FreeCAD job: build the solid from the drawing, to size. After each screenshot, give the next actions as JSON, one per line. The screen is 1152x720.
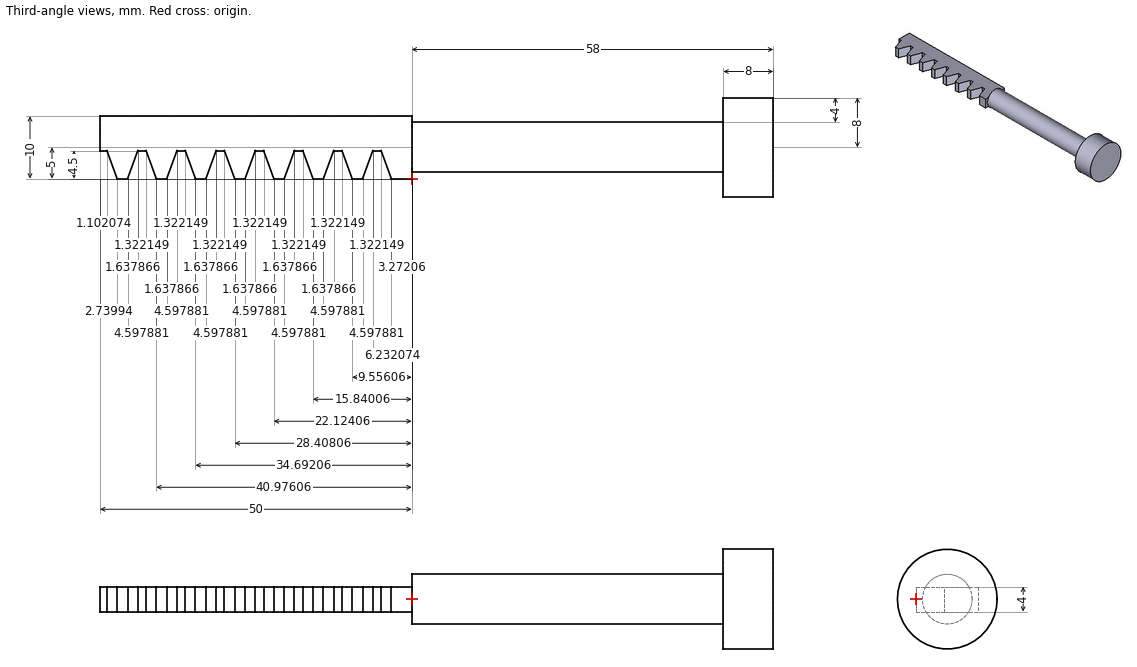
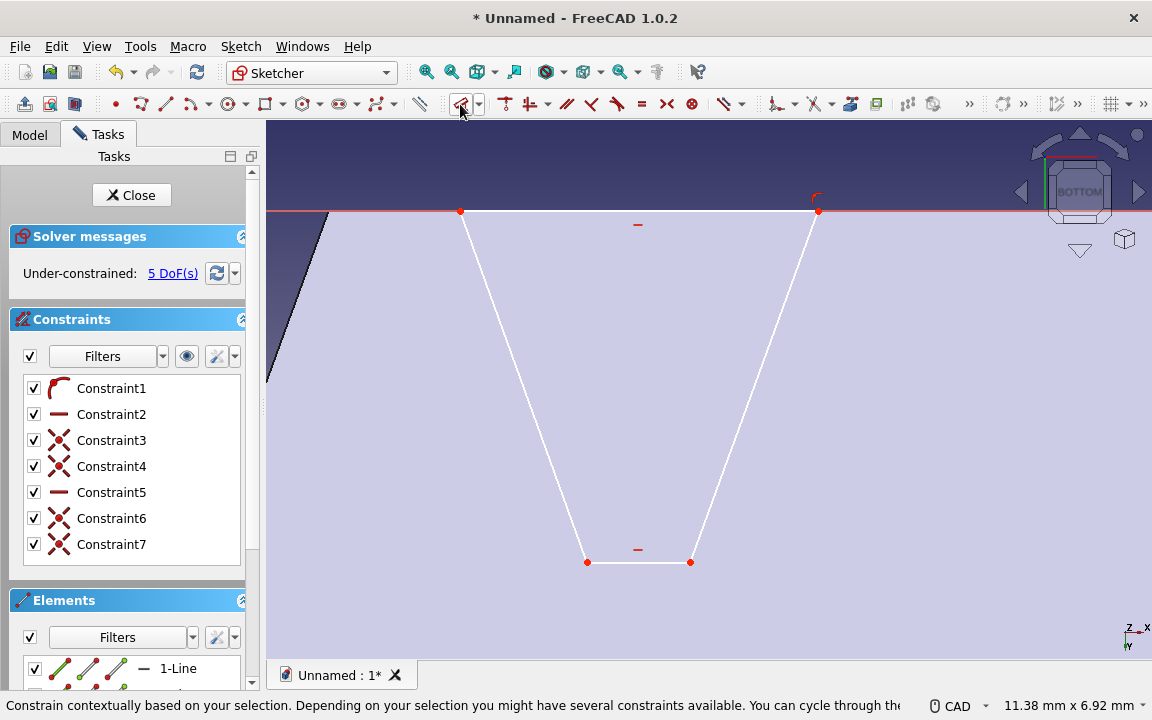
{"action": "left_click", "coordinate": [587, 563]}
{"action": "left_click", "coordinate": [553, 387]}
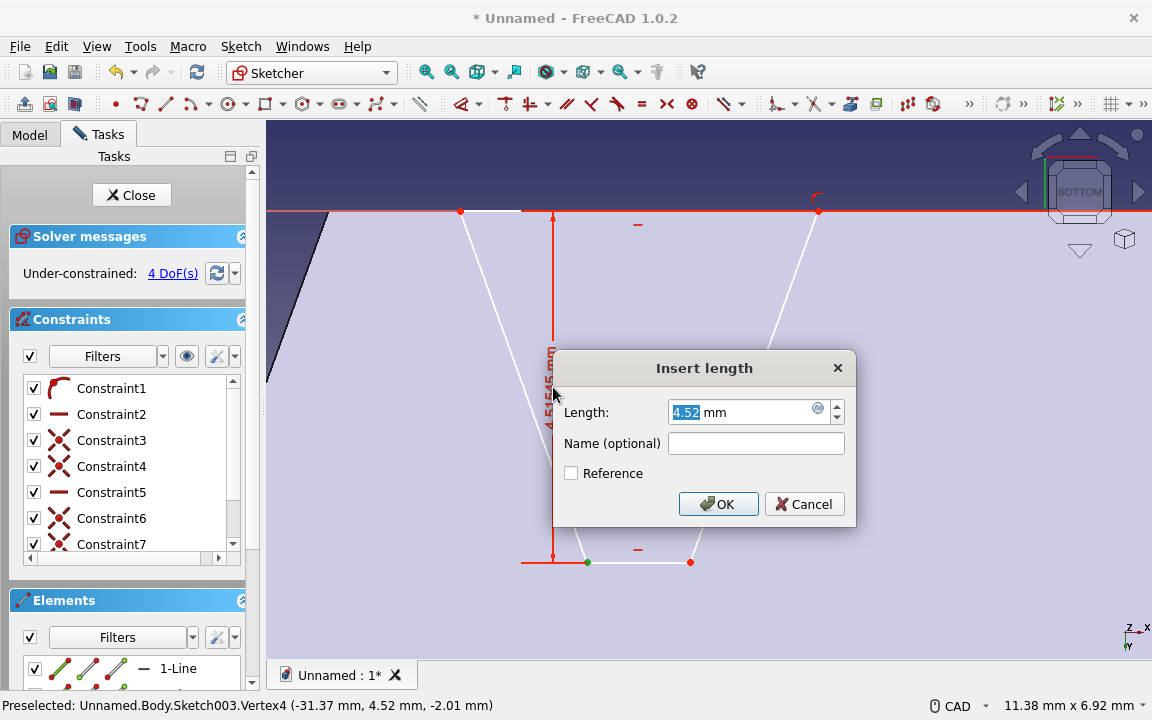
{"action": "type", "text": "4.5"}
{"action": "key", "text": "Return"}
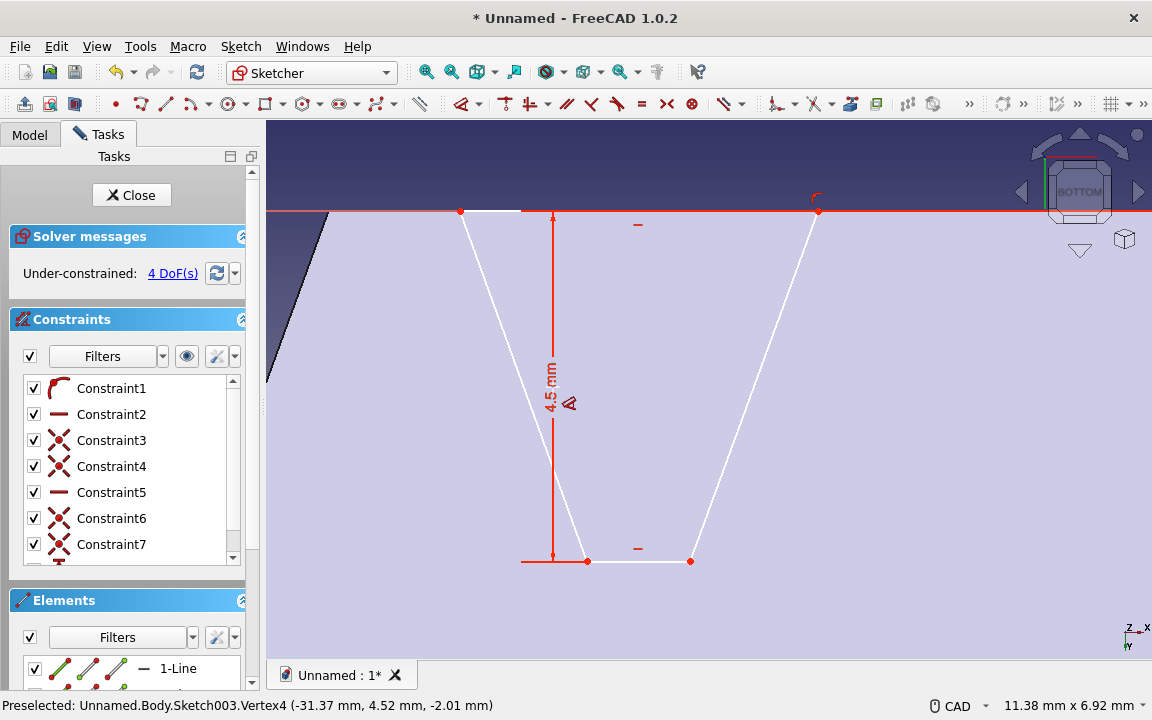
{"action": "left_click", "coordinate": [711, 211]}
{"action": "left_click", "coordinate": [639, 177]}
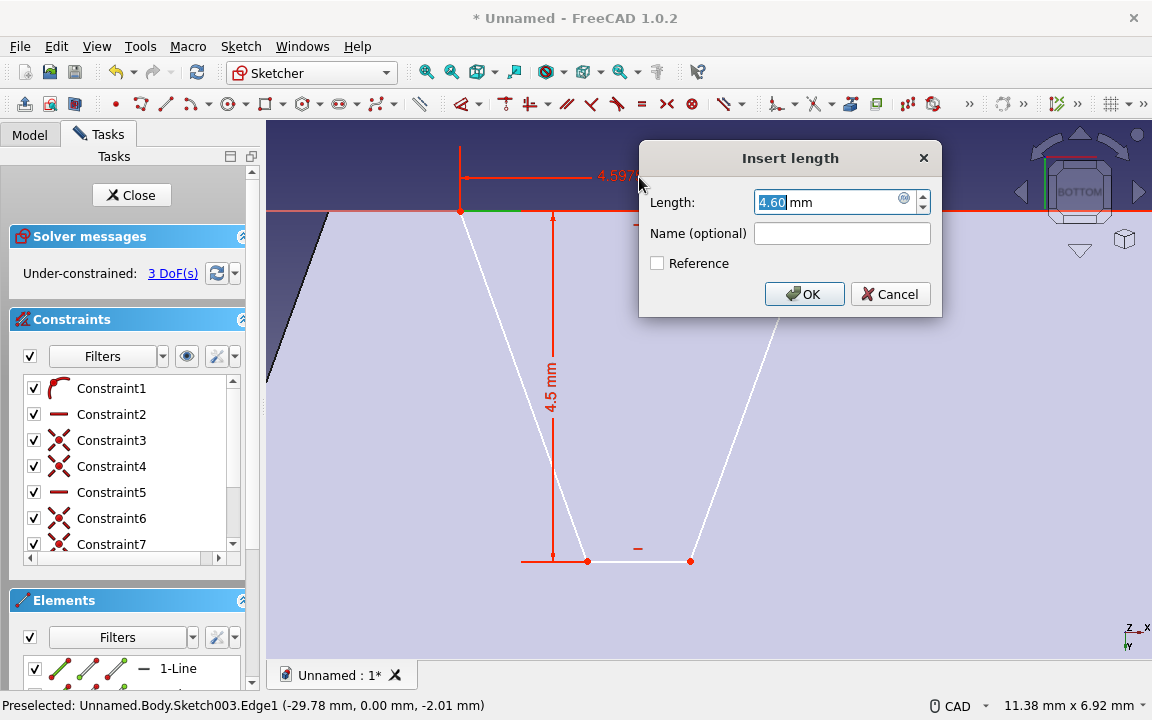
{"action": "type", "text": "4.597881"}
{"action": "key", "text": "Return"}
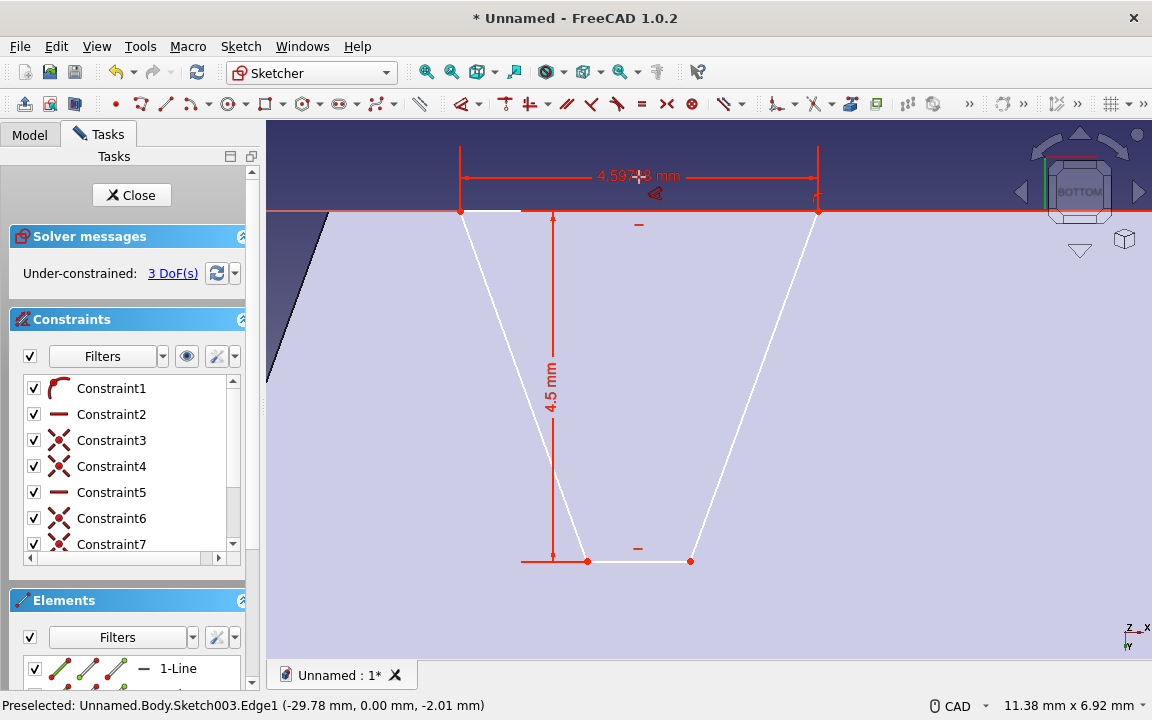
{"action": "left_click", "coordinate": [618, 562]}
{"action": "left_click", "coordinate": [638, 596]}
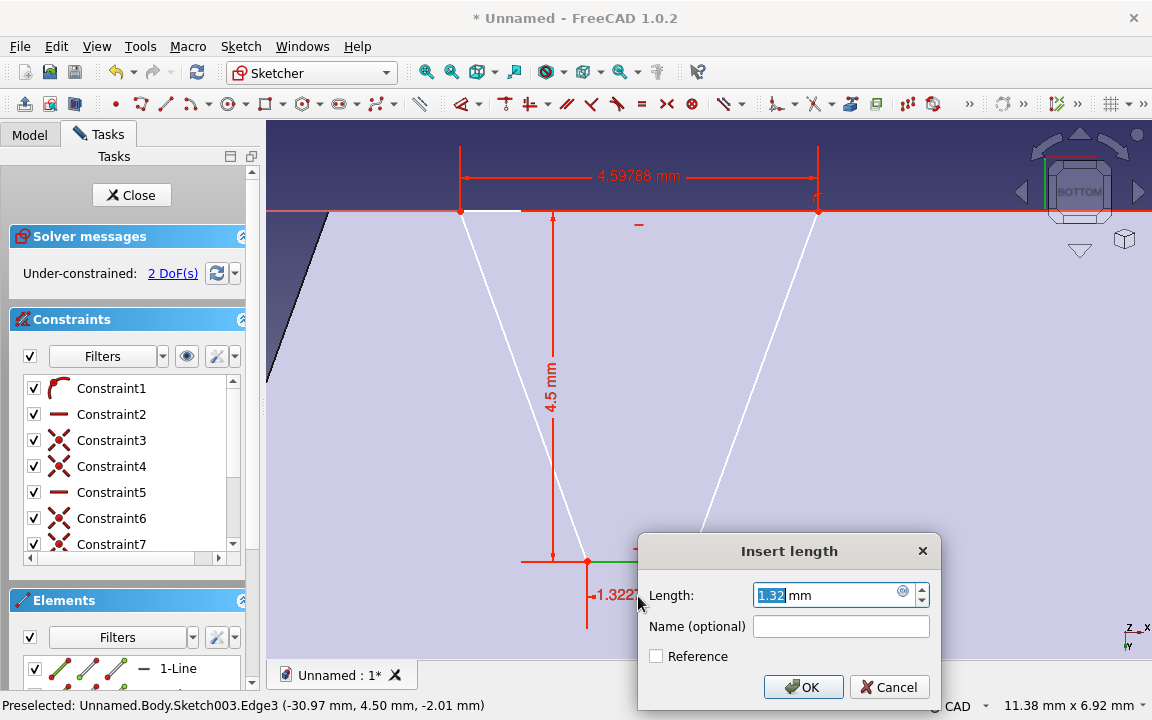
{"action": "type", "text": "1.322149"}
{"action": "key", "text": "Return"}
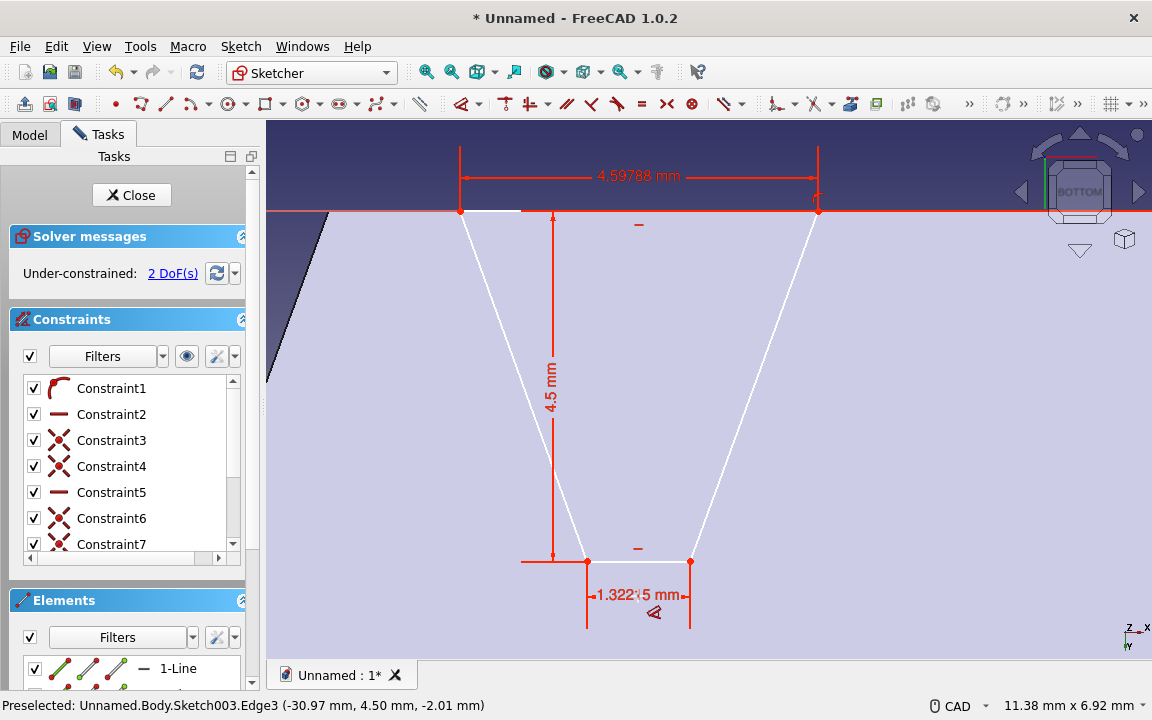
{"action": "left_click", "coordinate": [818, 211]}
{"action": "left_click", "coordinate": [903, 177]}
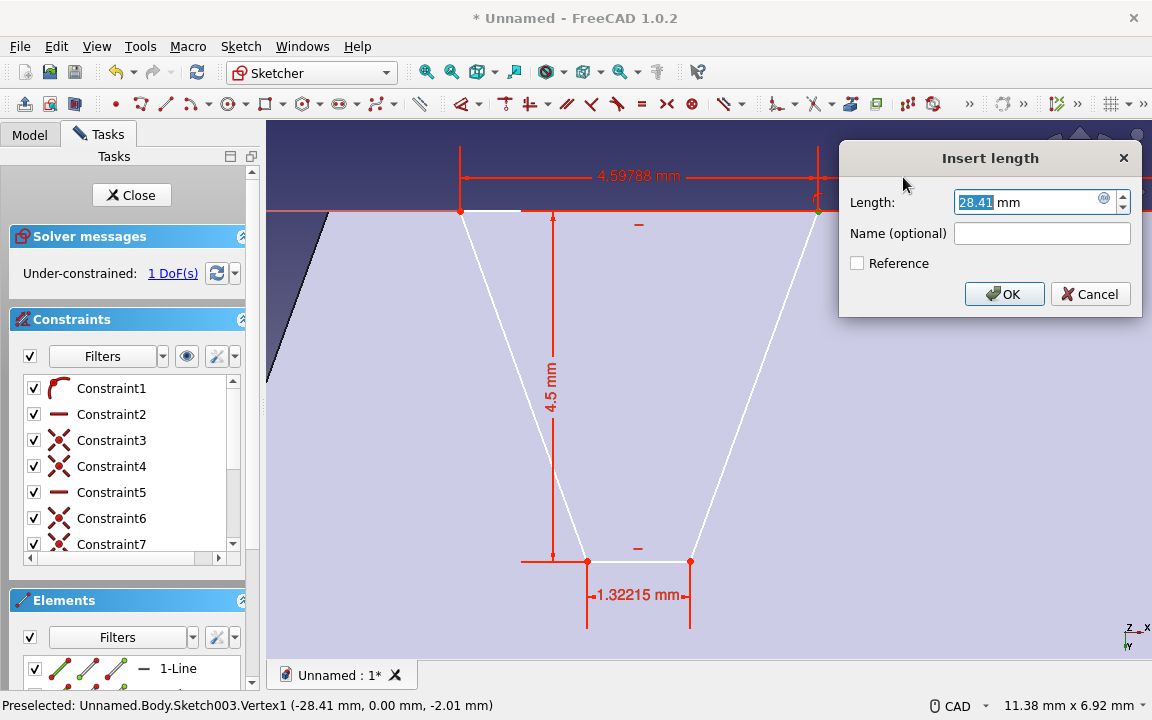
{"action": "type", "text": "28.40806"}
{"action": "key", "text": "Return"}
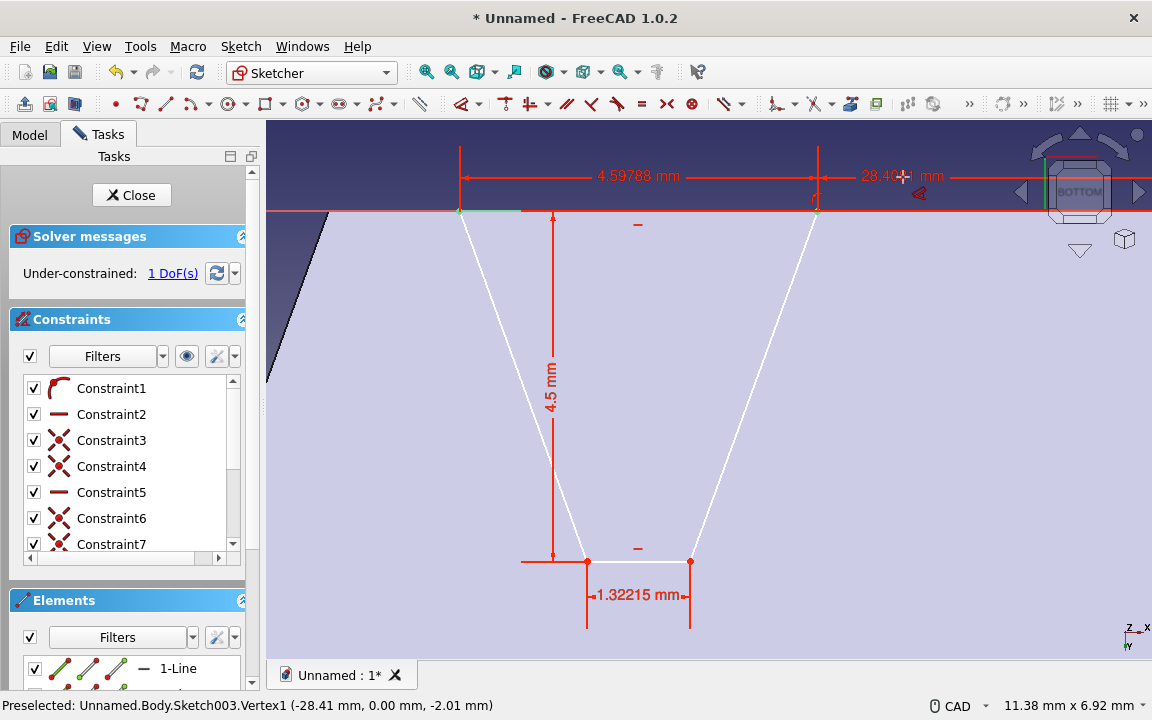
{"action": "left_click", "coordinate": [498, 317]}
{"action": "left_click", "coordinate": [523, 596]}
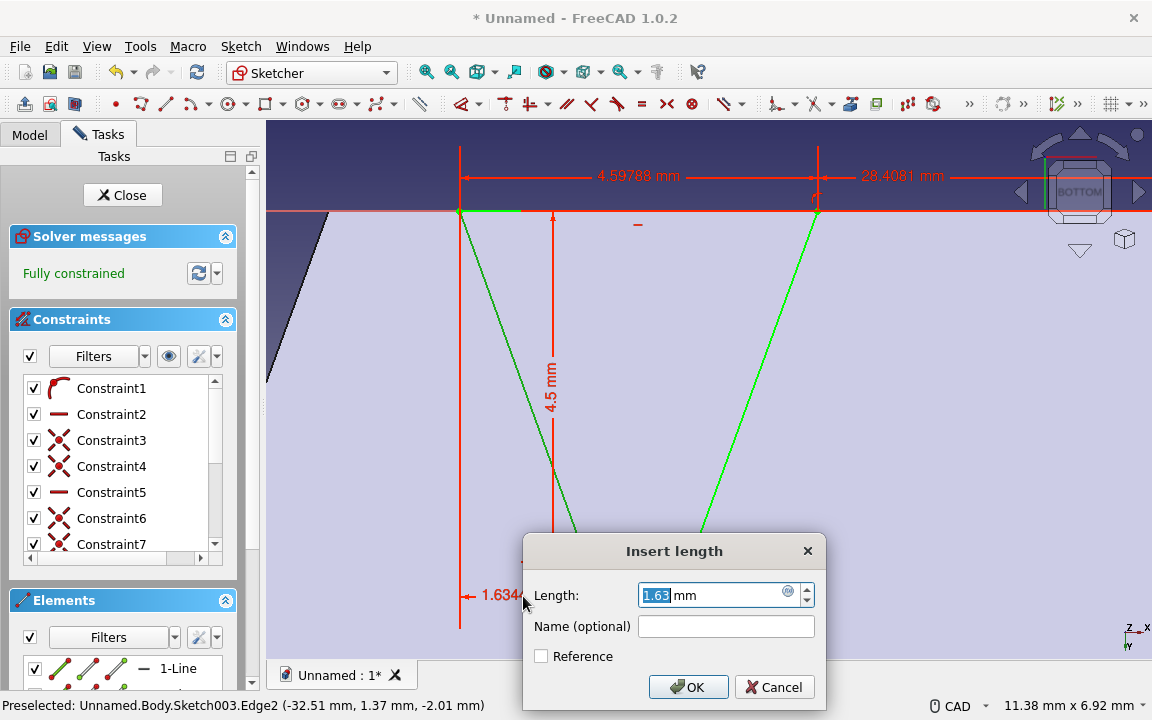
{"action": "type", "text": "1.637866"}
{"action": "key", "text": "Return"}
{"action": "key", "text": "Escape"}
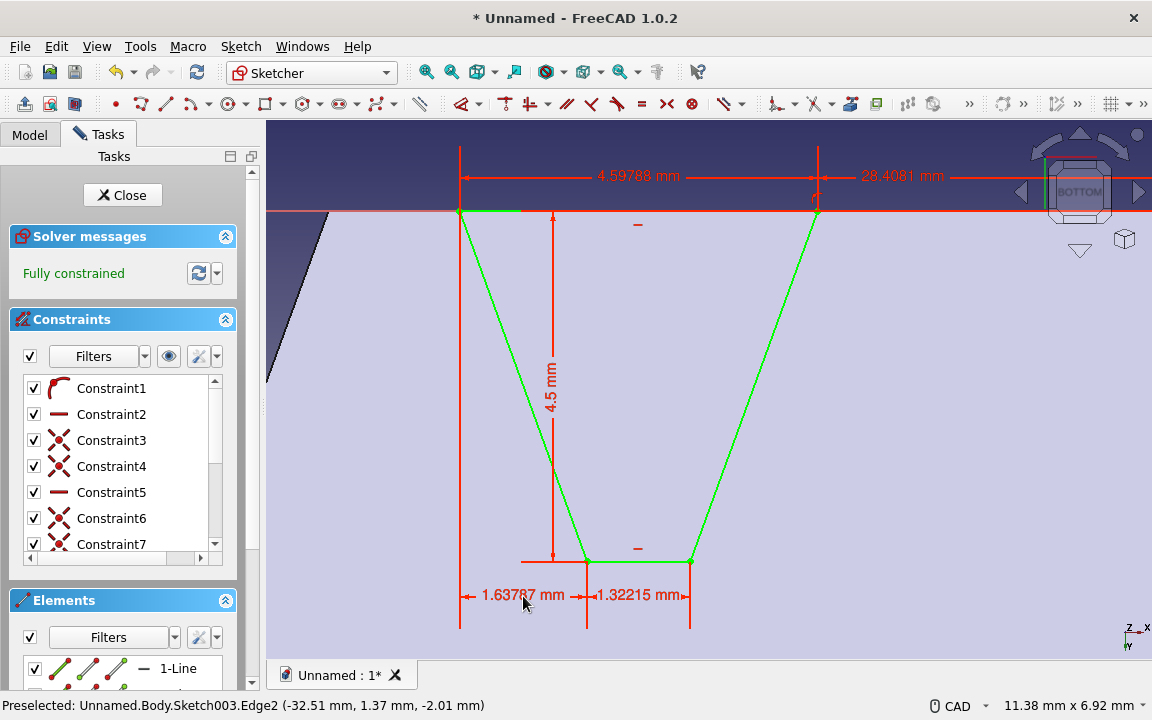
{"action": "left_click", "coordinate": [123, 195]}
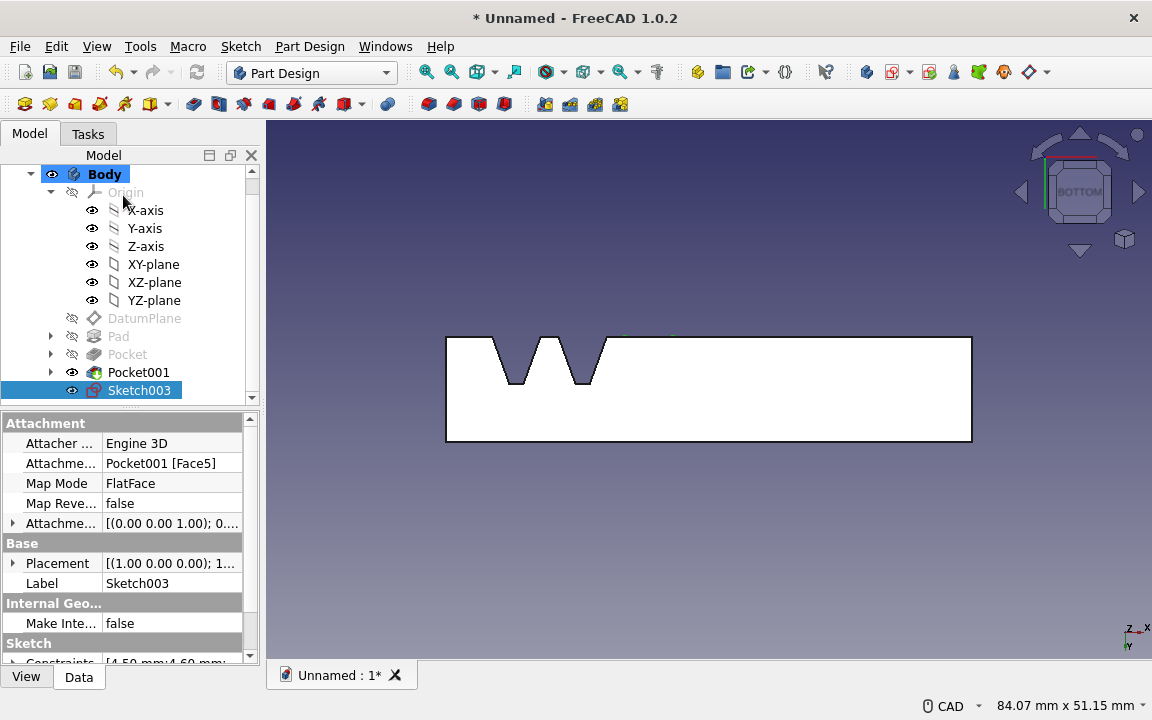
{"action": "left_click", "coordinate": [194, 104]}